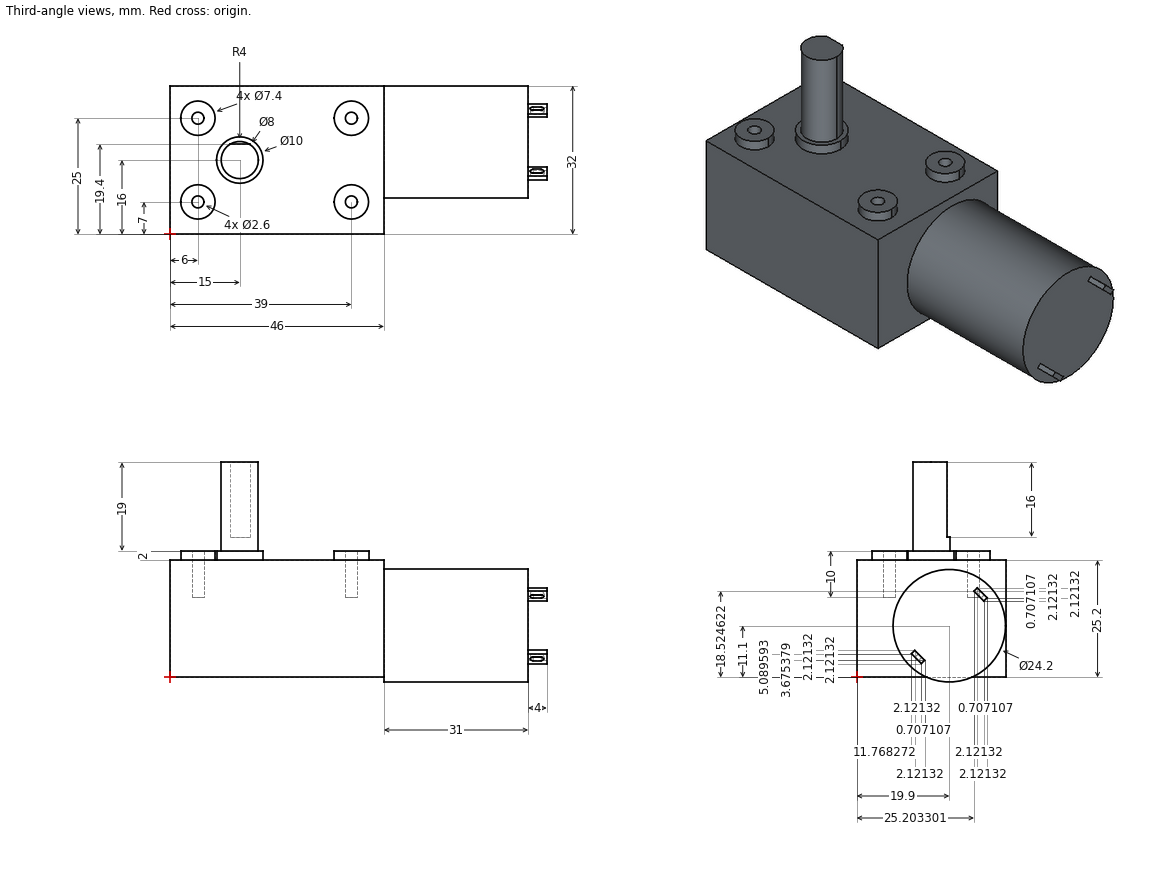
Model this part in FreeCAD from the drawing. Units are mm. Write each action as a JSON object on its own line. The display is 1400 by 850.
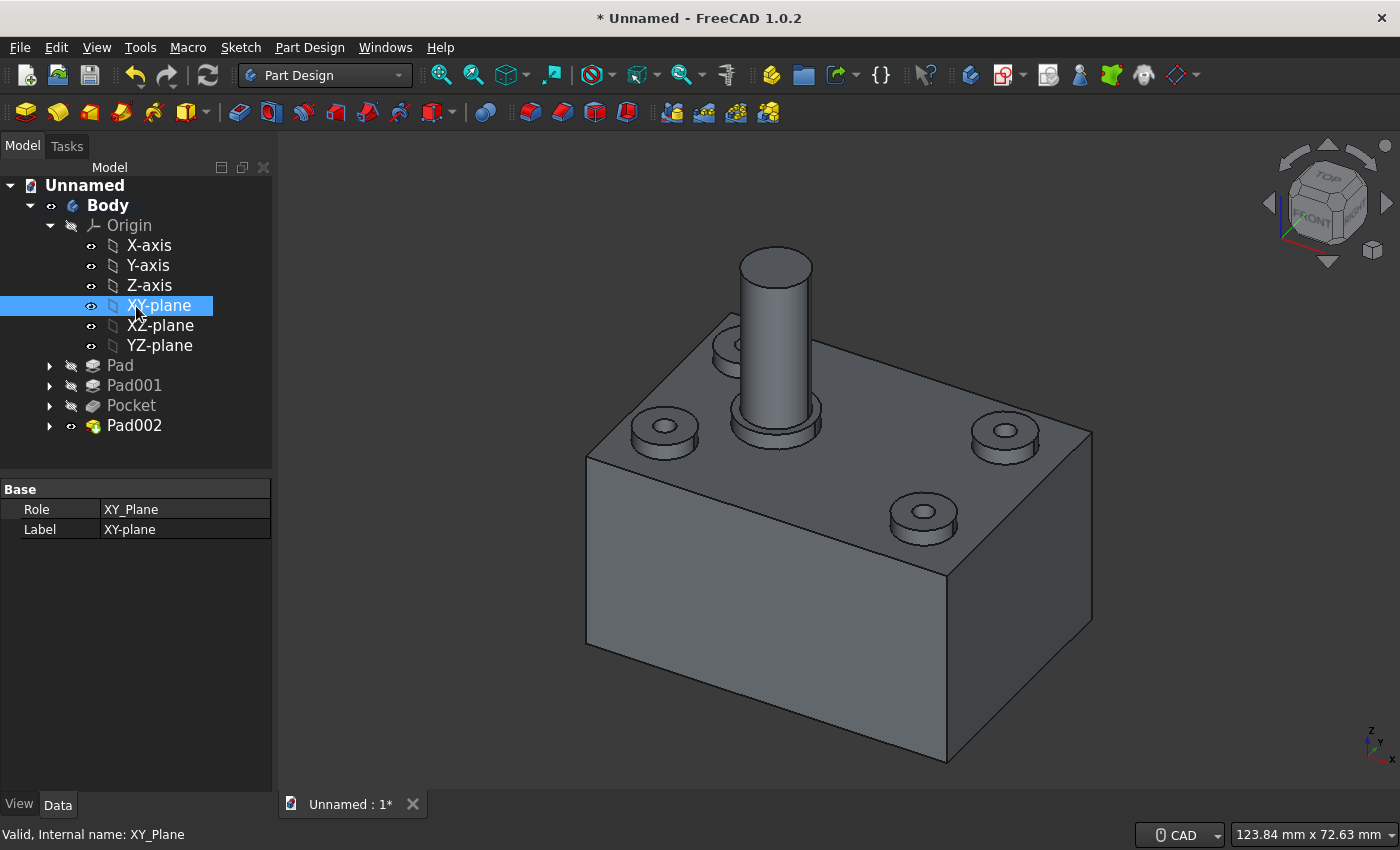
{"action": "left_click", "coordinate": [1176, 76]}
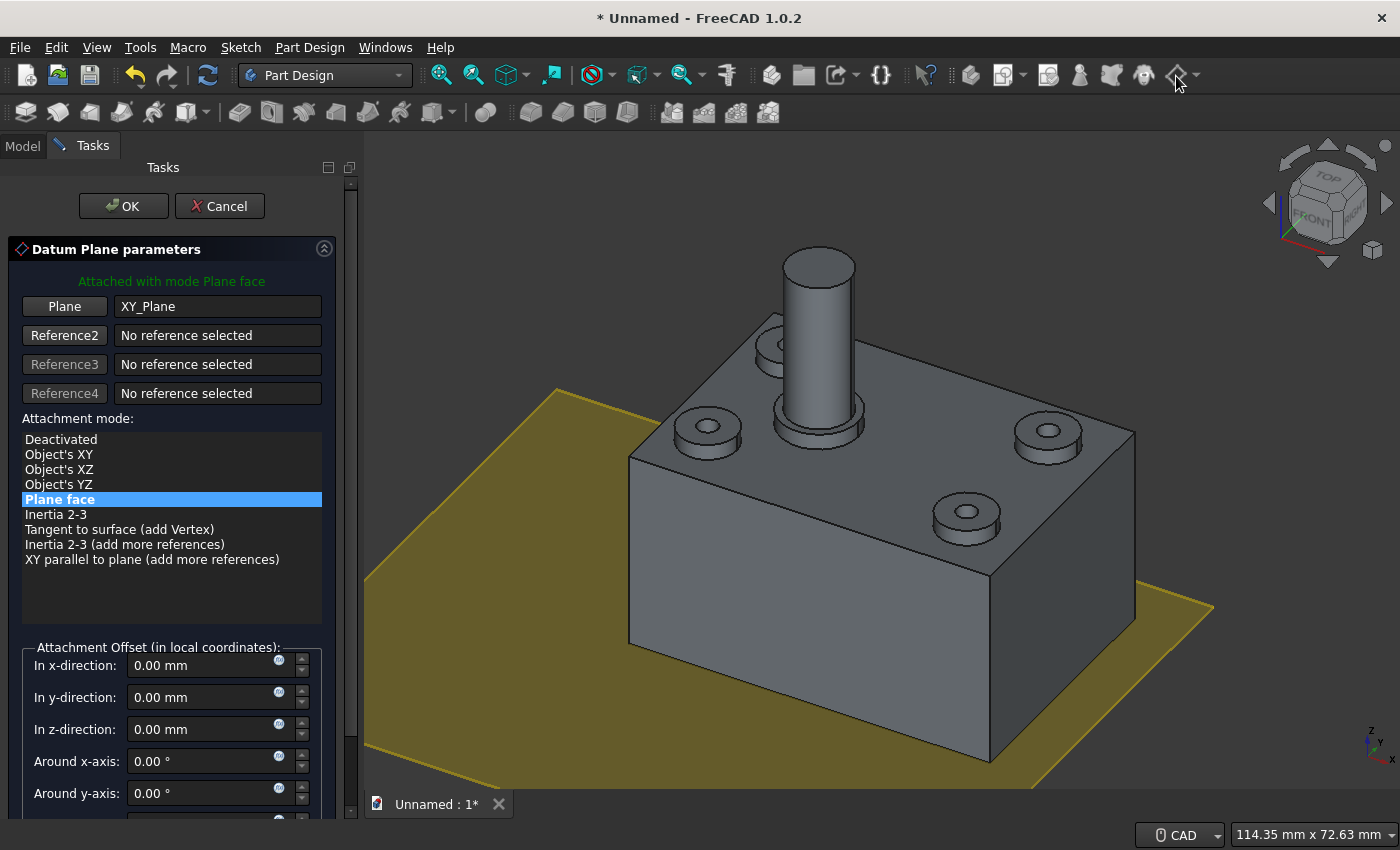
{"action": "triple_click", "coordinate": [210, 729]}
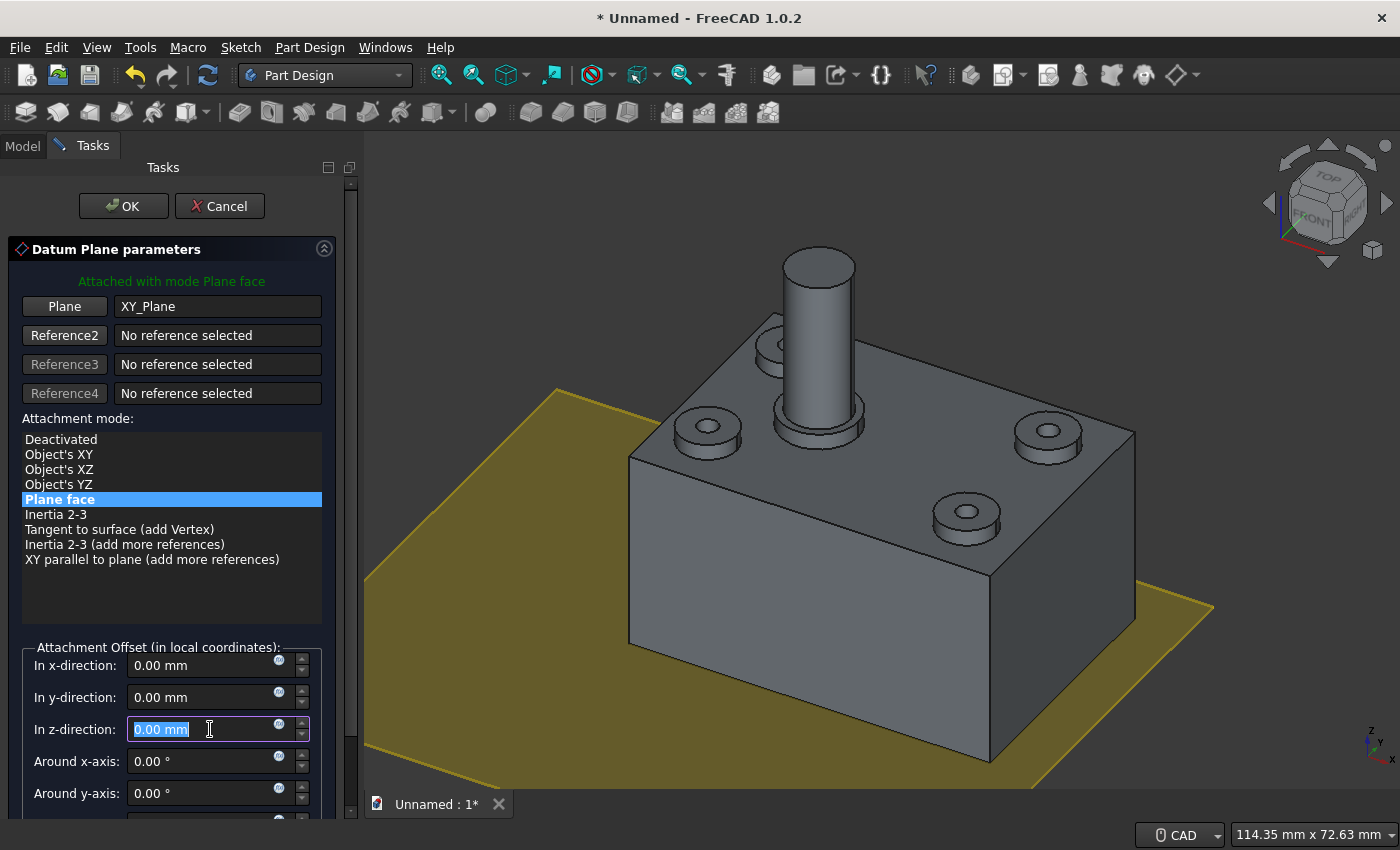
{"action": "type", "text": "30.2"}
{"action": "key", "text": "Tab"}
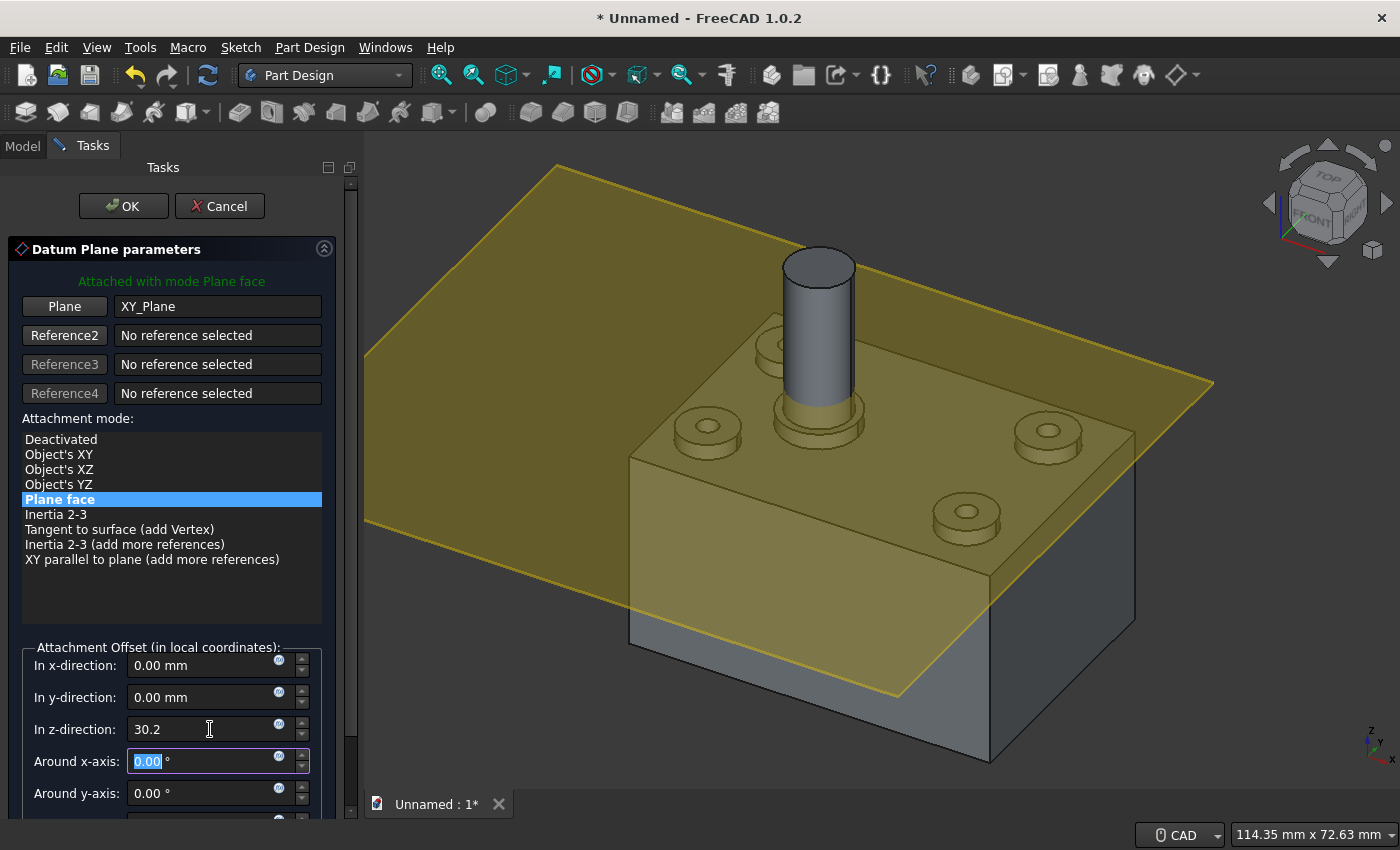
{"action": "left_click", "coordinate": [124, 206]}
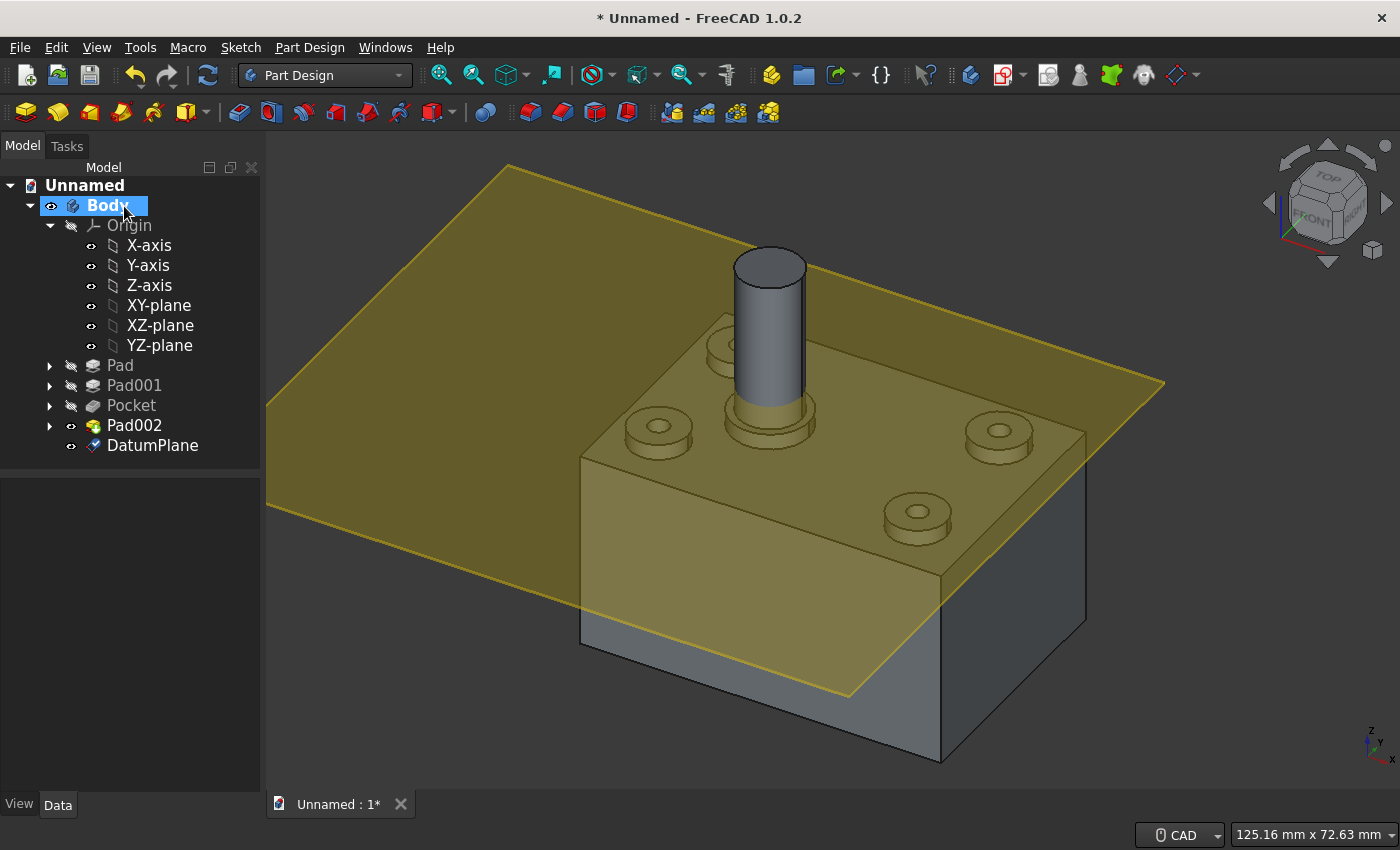
{"action": "left_click", "coordinate": [116, 446]}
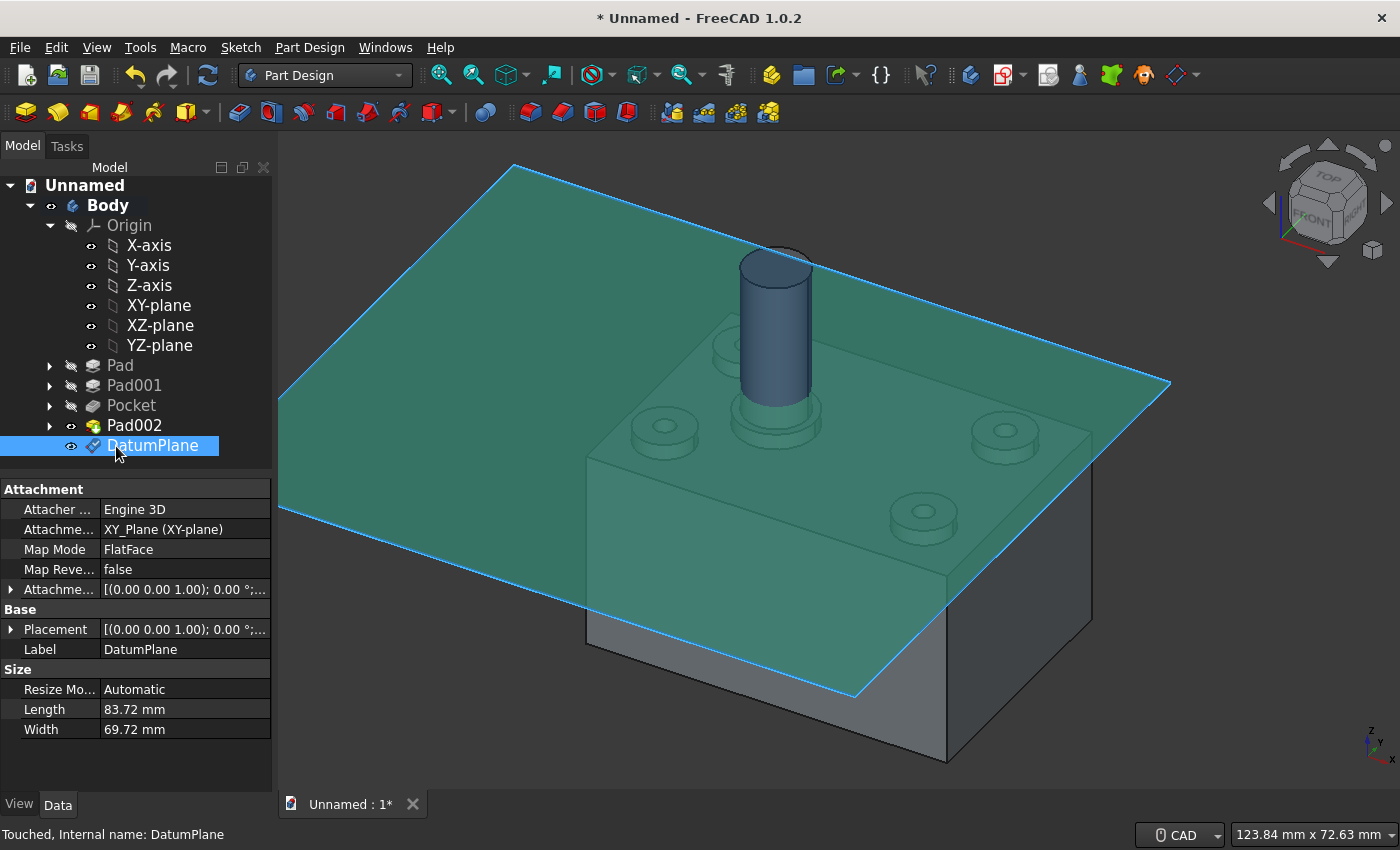
{"action": "left_click", "coordinate": [1004, 76]}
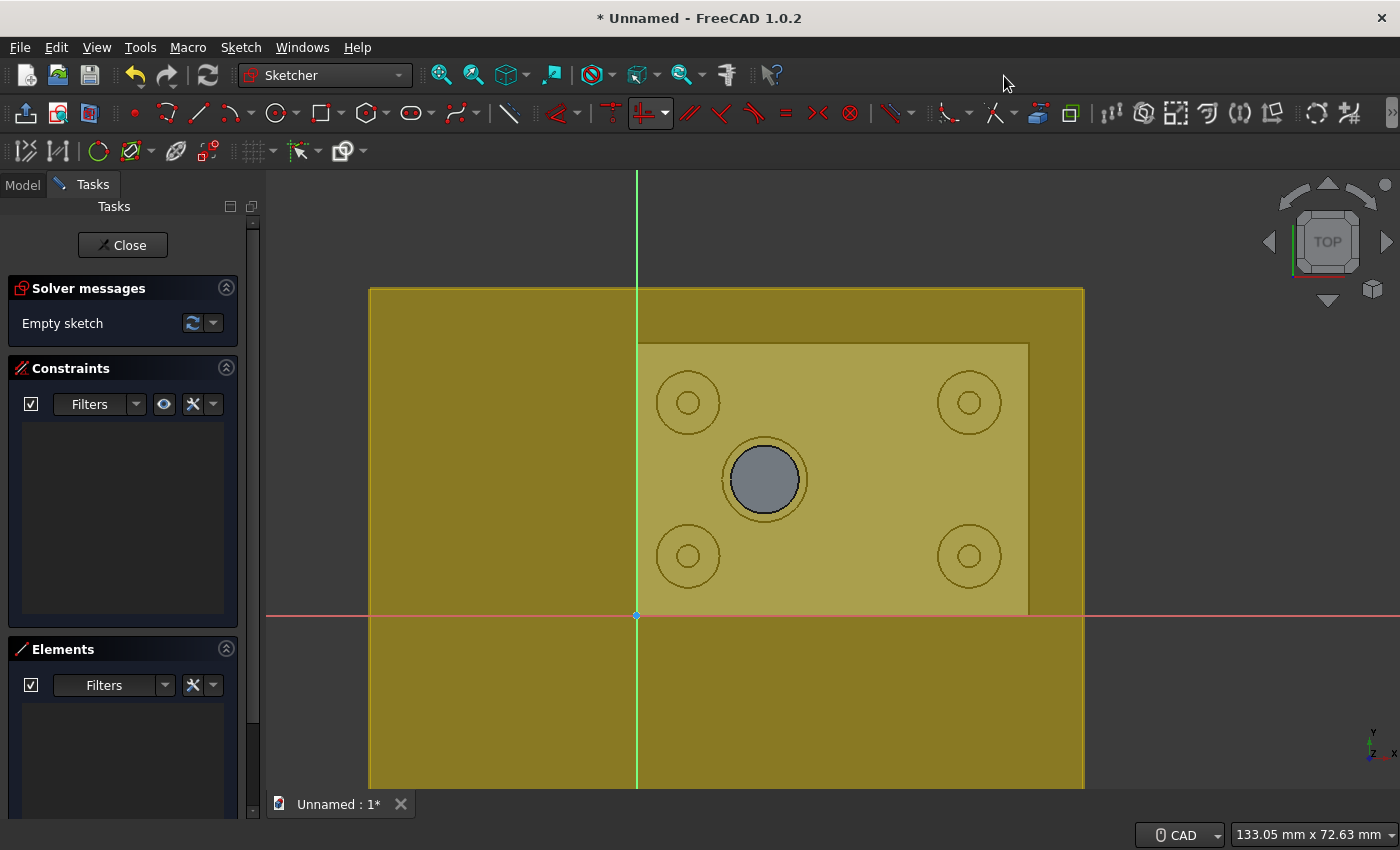
{"action": "left_click", "coordinate": [90, 114]}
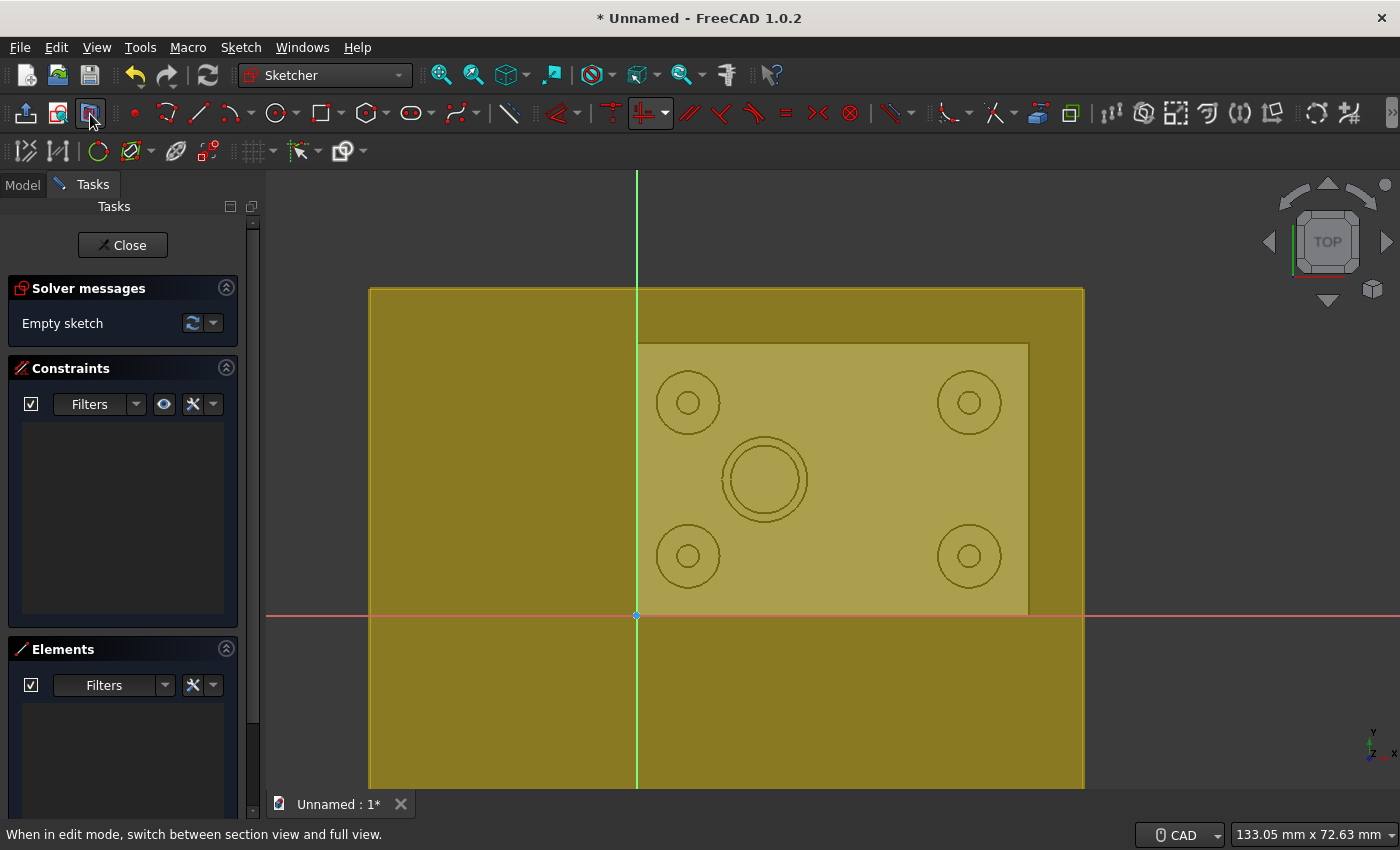
{"action": "scroll", "coordinate": [765, 446], "scroll_direction": "up", "scroll_amount": 15}